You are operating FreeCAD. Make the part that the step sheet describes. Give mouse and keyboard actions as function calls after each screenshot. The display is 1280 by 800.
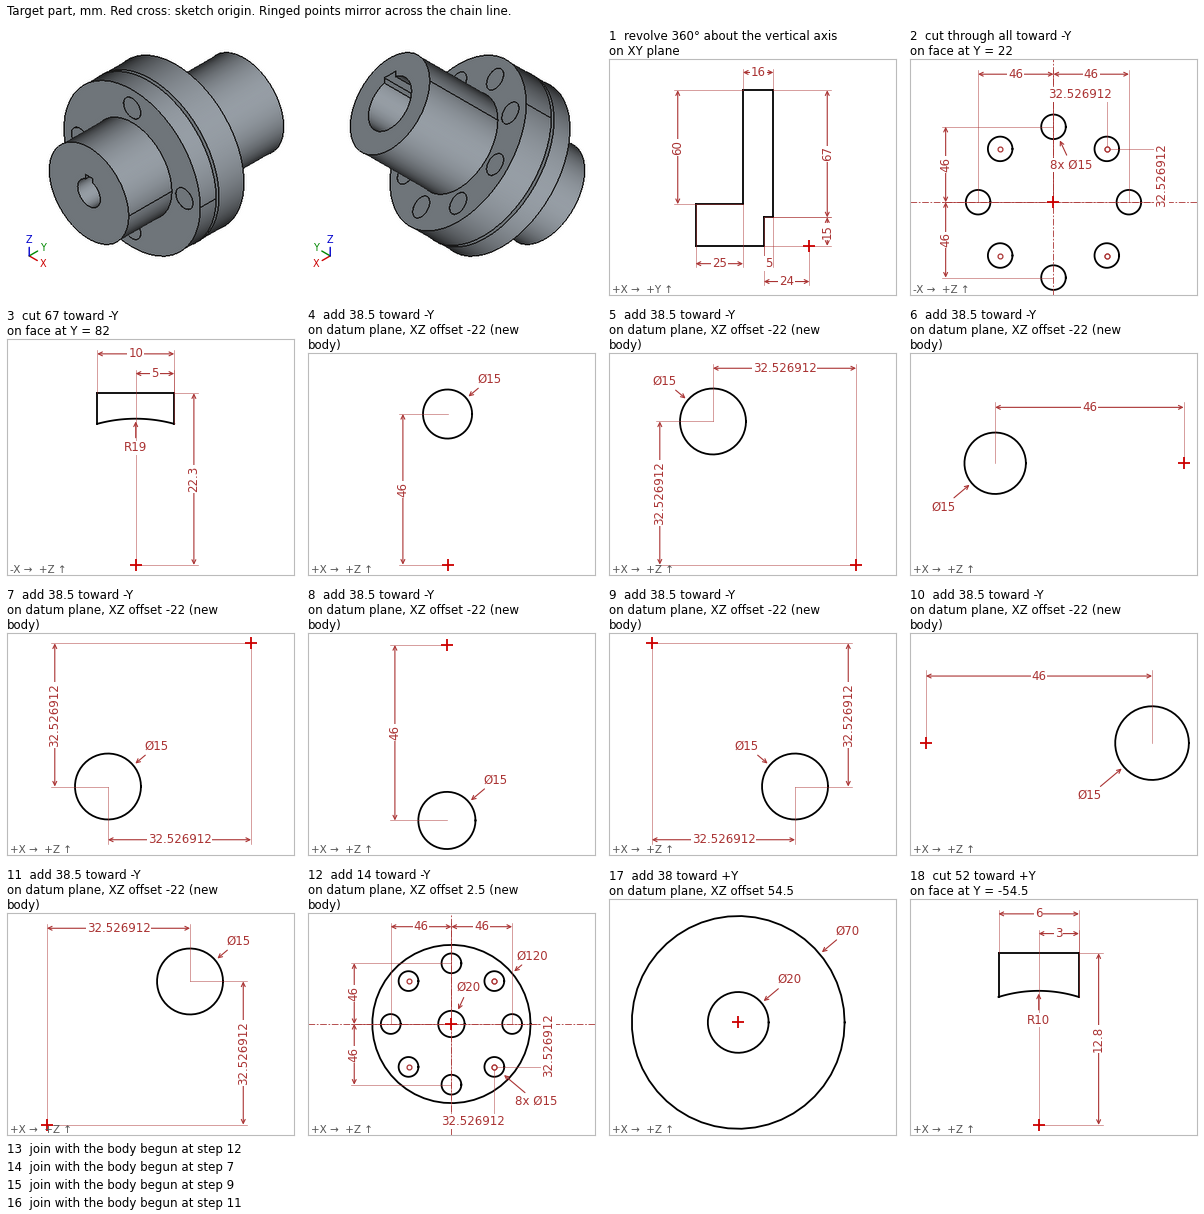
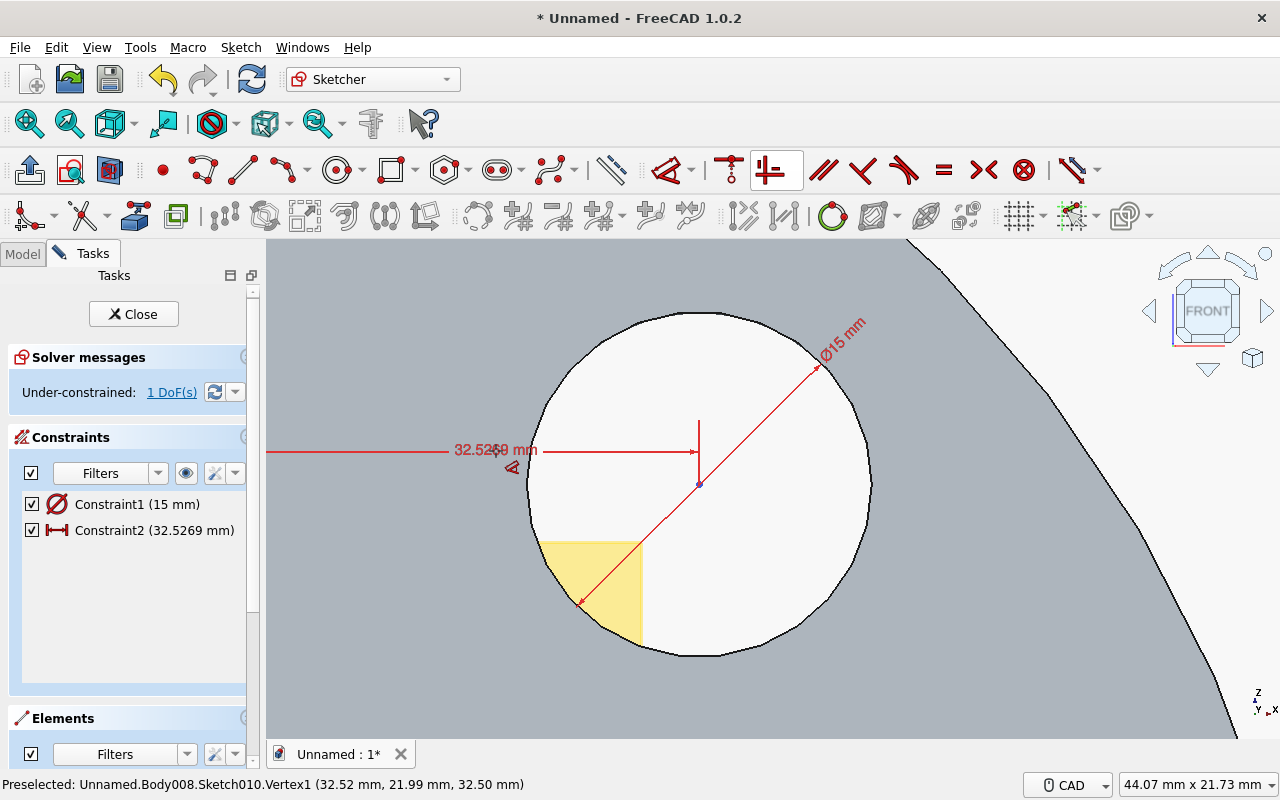
click(699, 485)
click(733, 598)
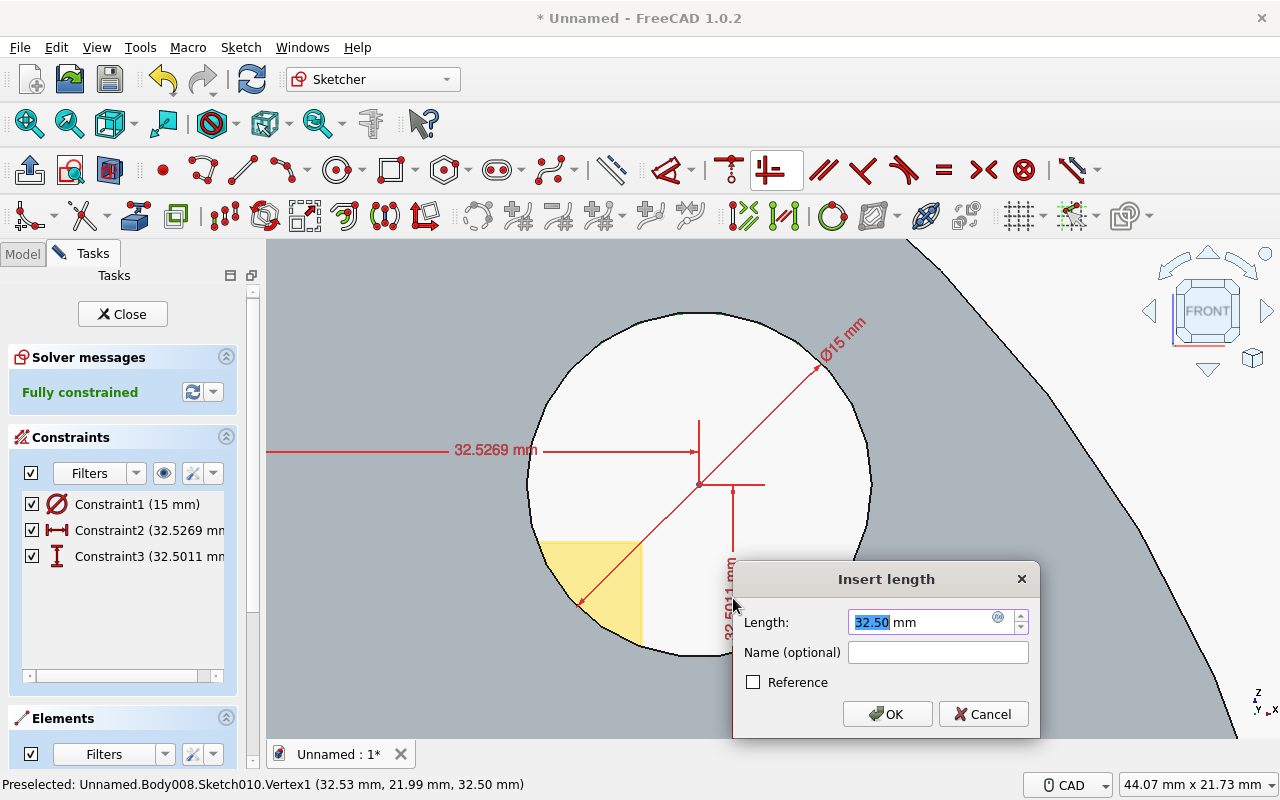
text(32.526912)
key(Return)
key(Escape)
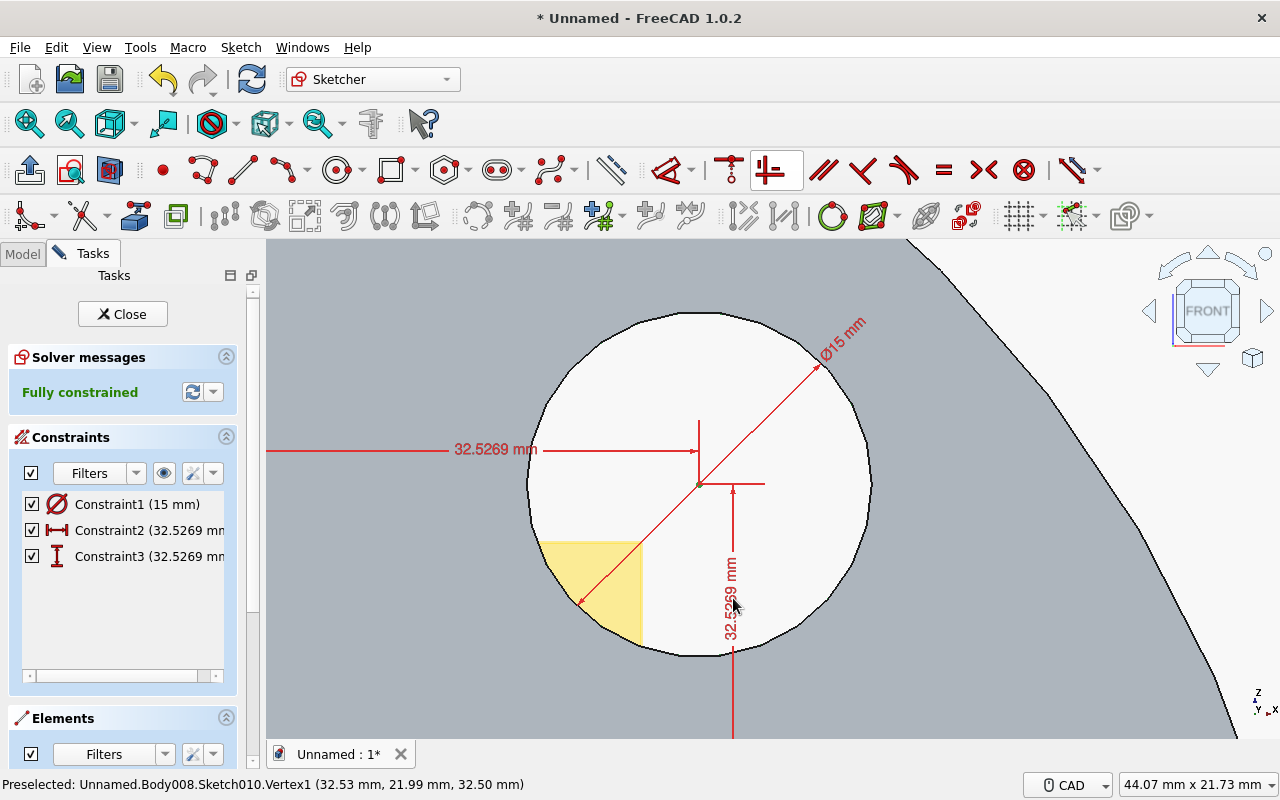
click(123, 314)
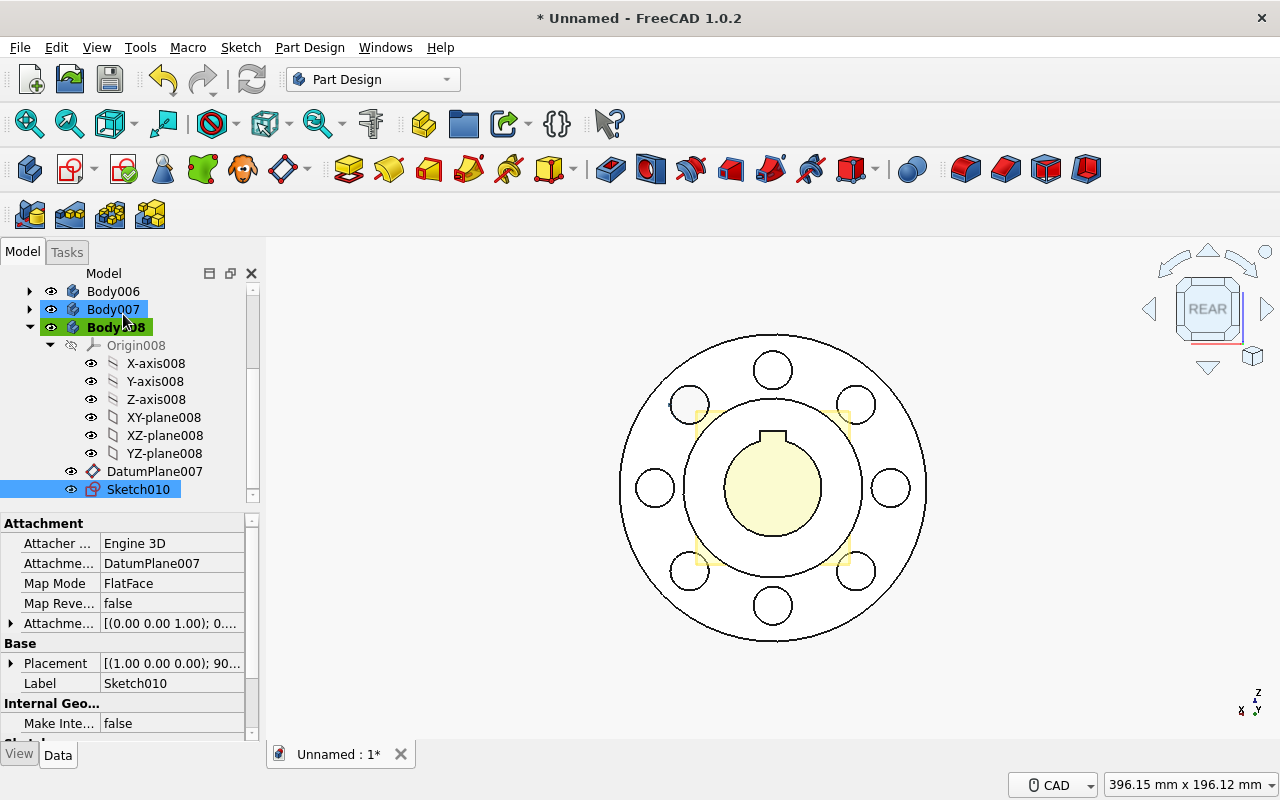
click(350, 170)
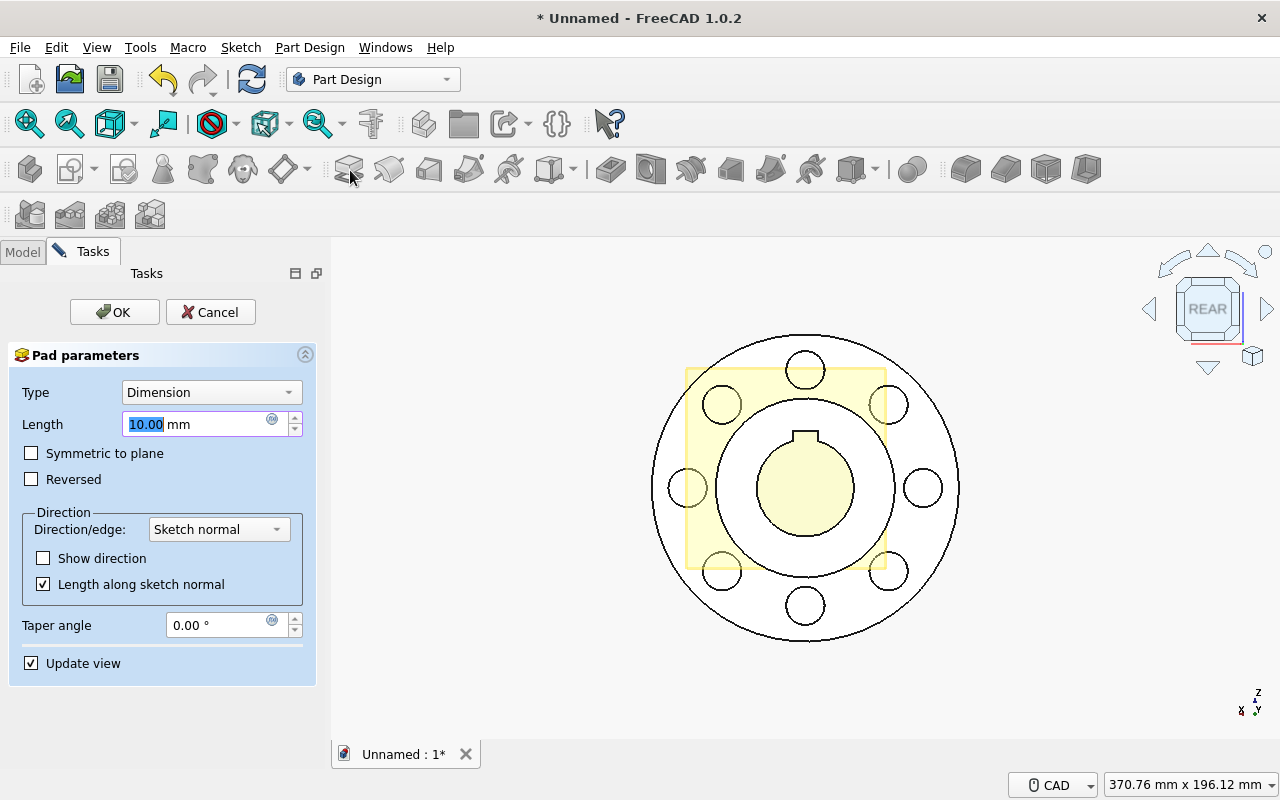
text(38.5)
key(Tab)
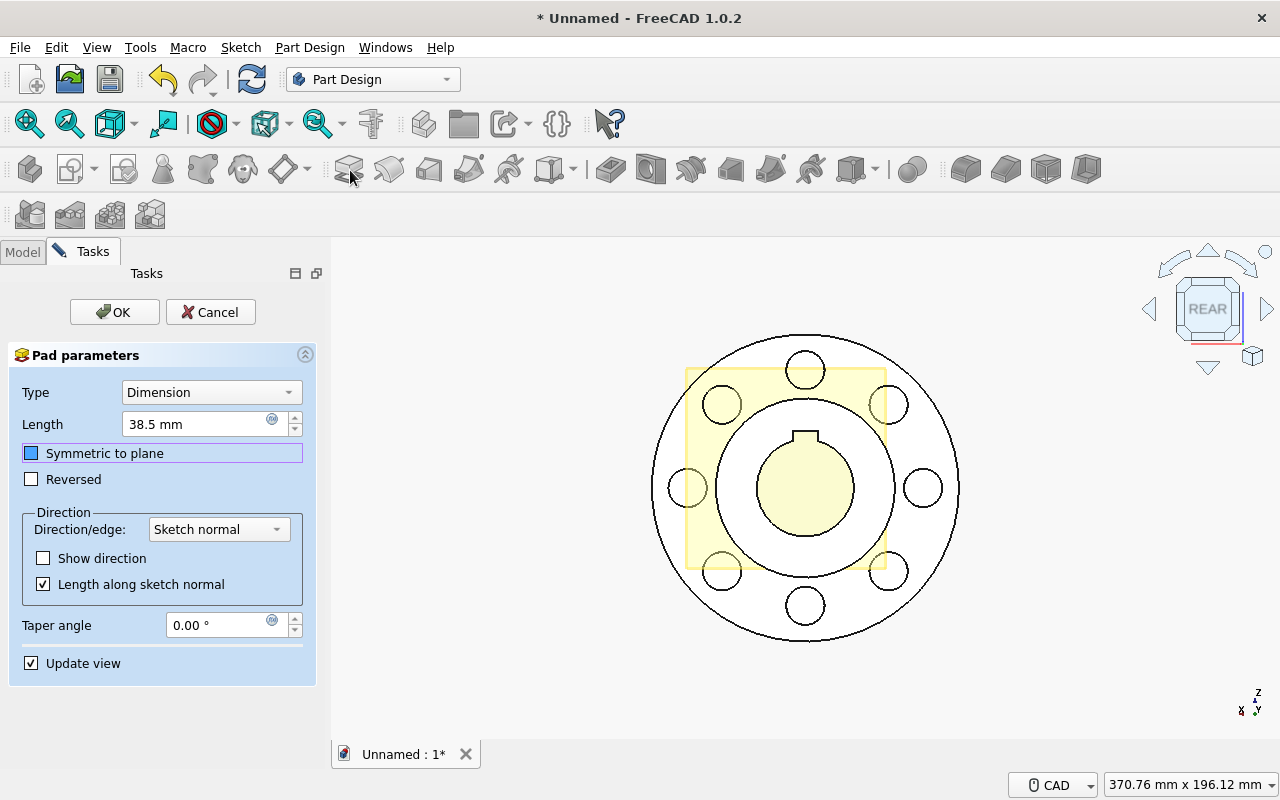
click(115, 312)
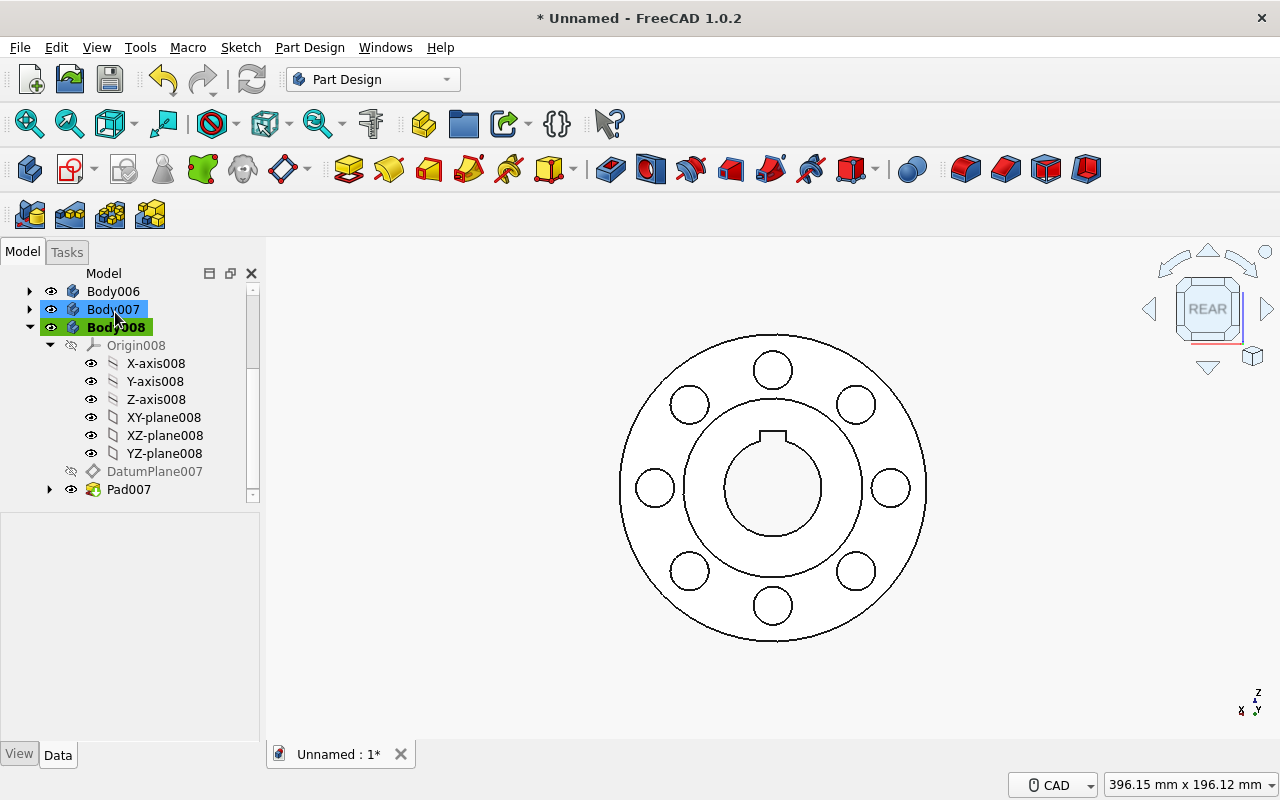
click(30, 124)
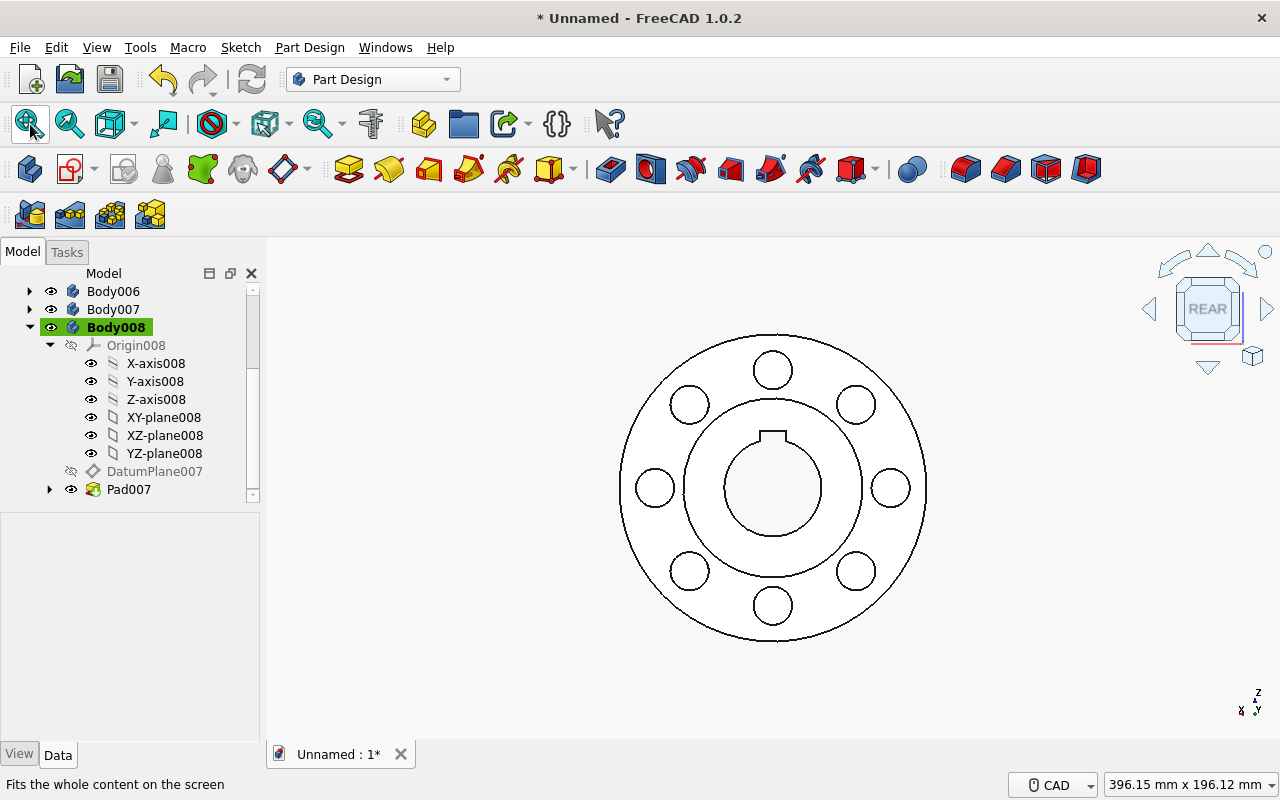
click(30, 170)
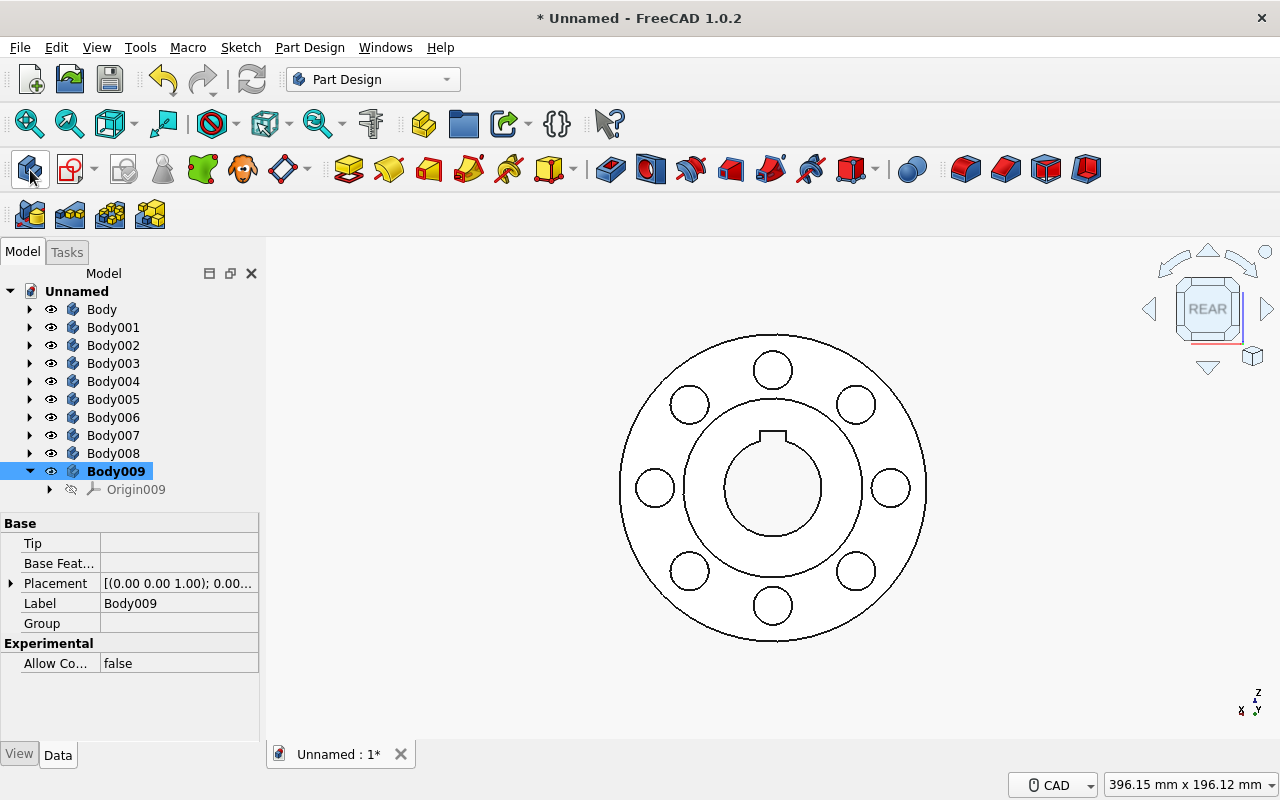
click(50, 489)